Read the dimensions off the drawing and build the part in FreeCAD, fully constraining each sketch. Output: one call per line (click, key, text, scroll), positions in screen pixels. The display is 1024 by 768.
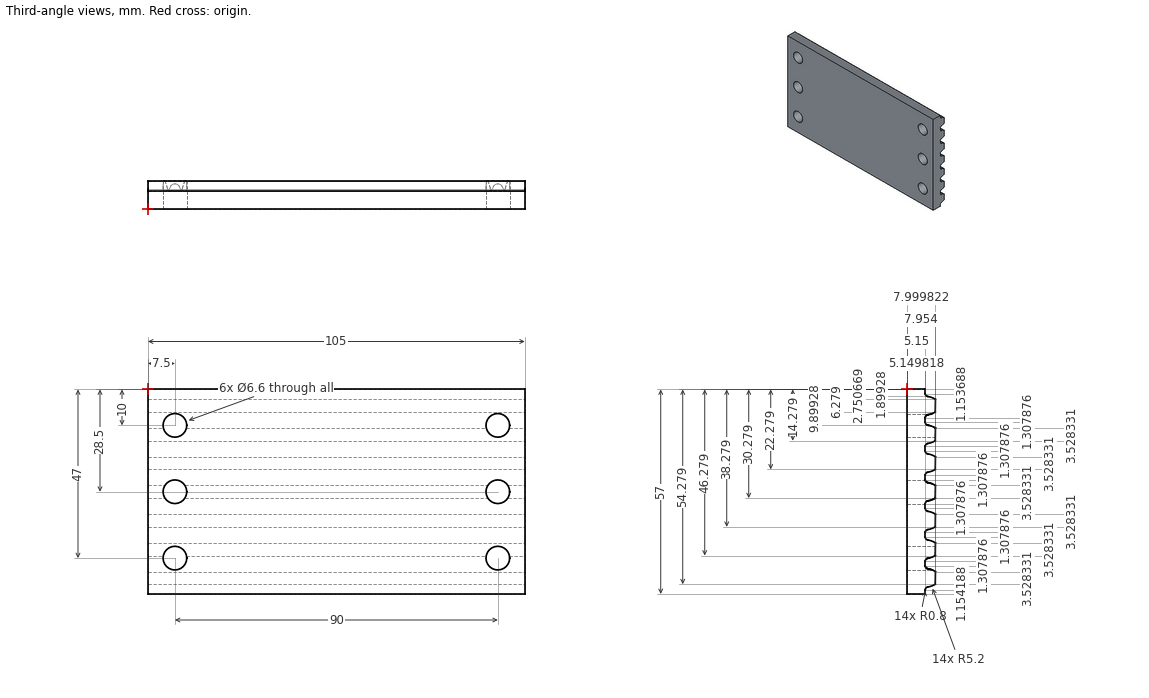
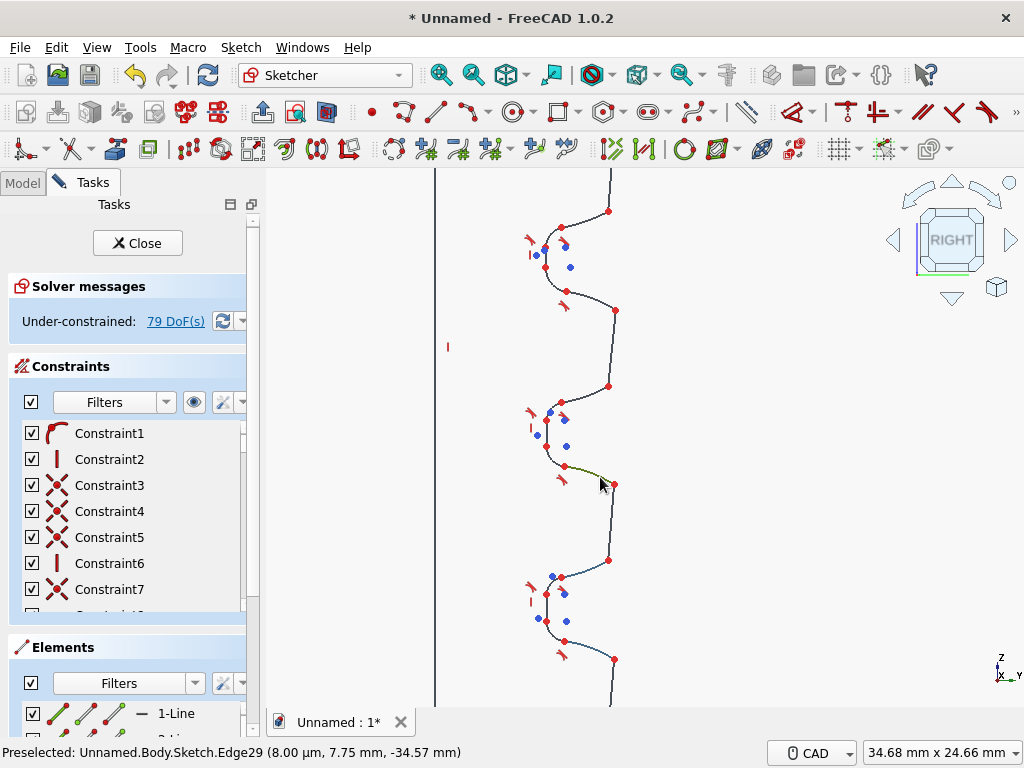
click(576, 400)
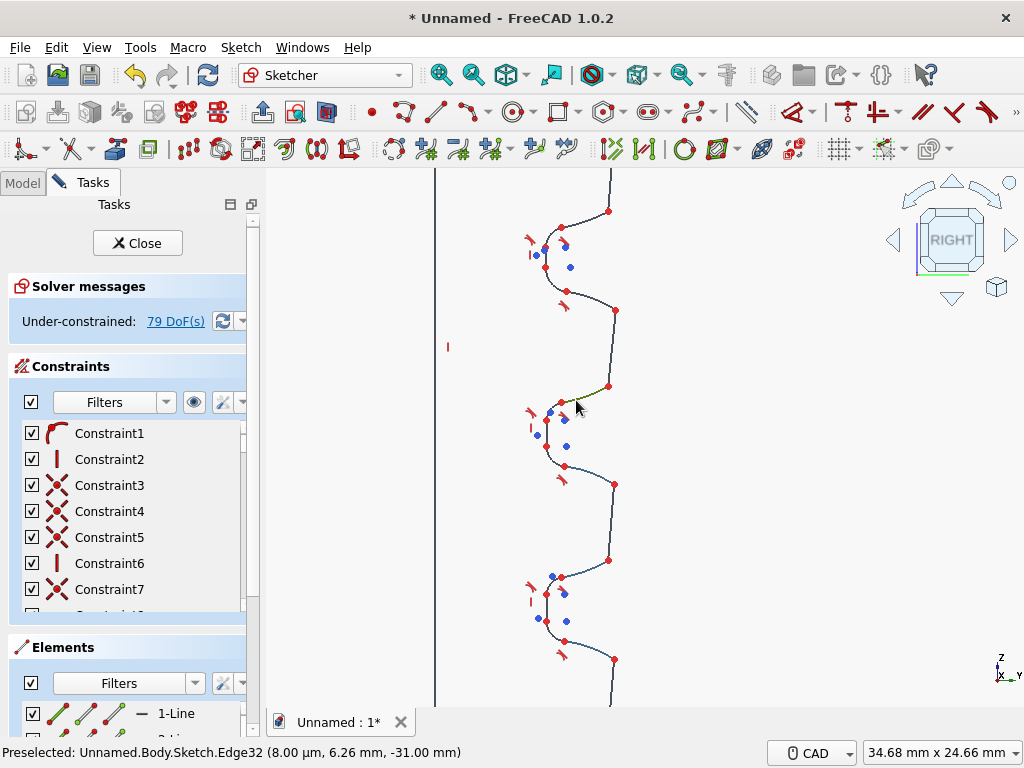
click(602, 302)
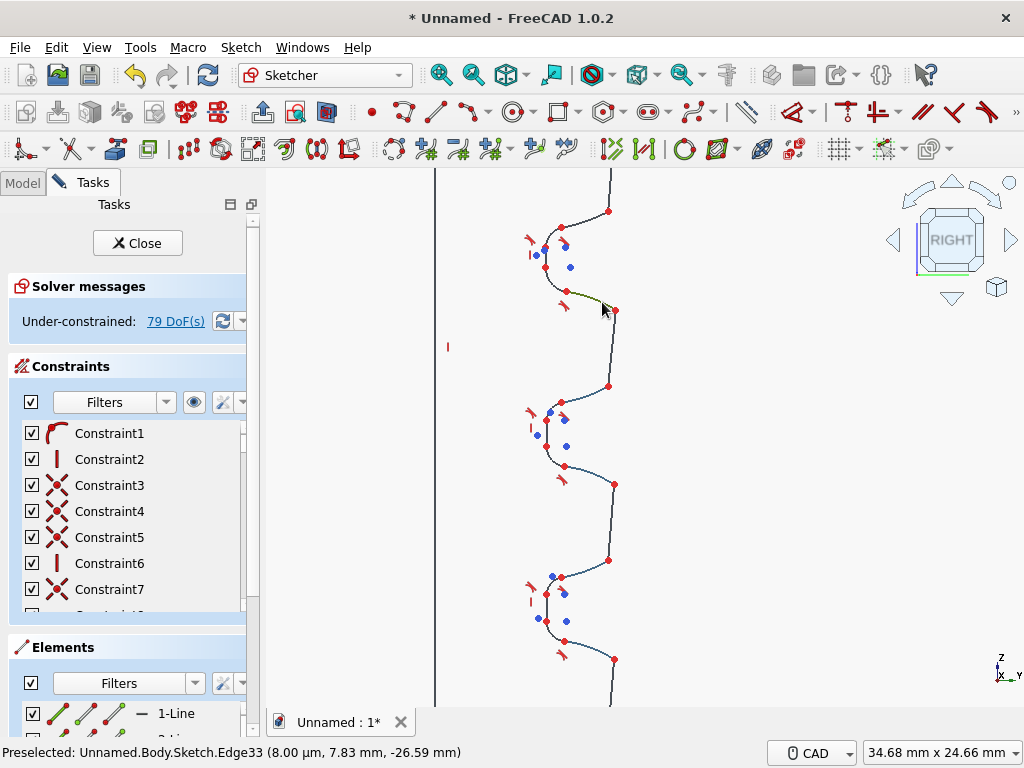
click(576, 224)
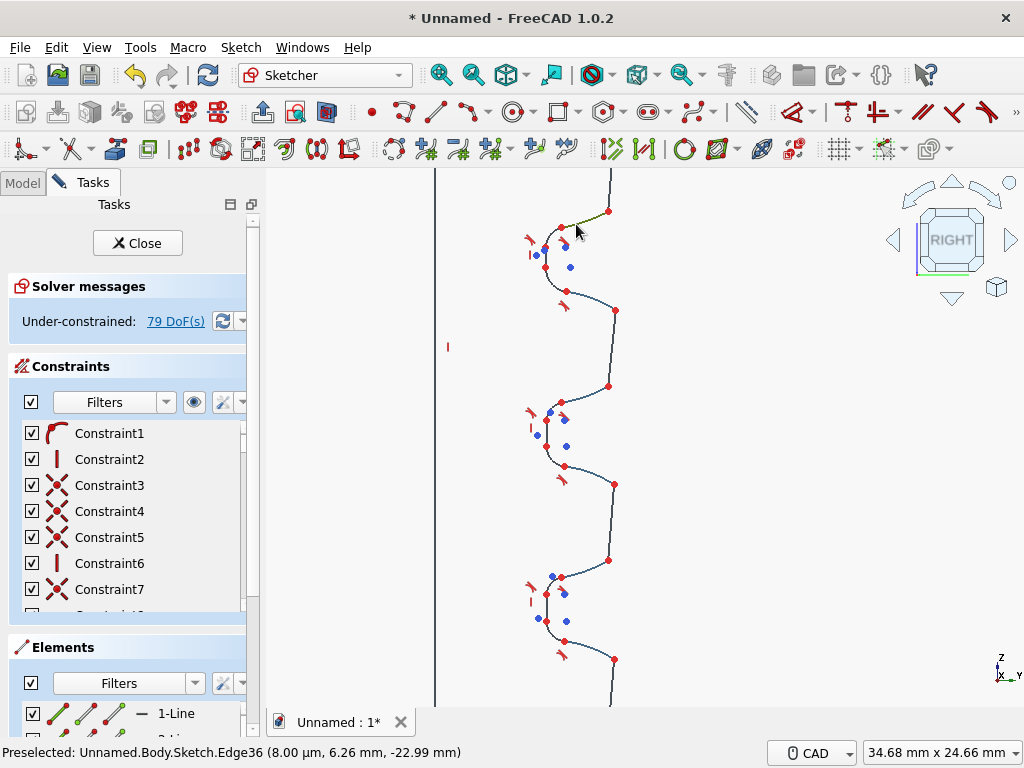
scroll(600, 477, down, 6)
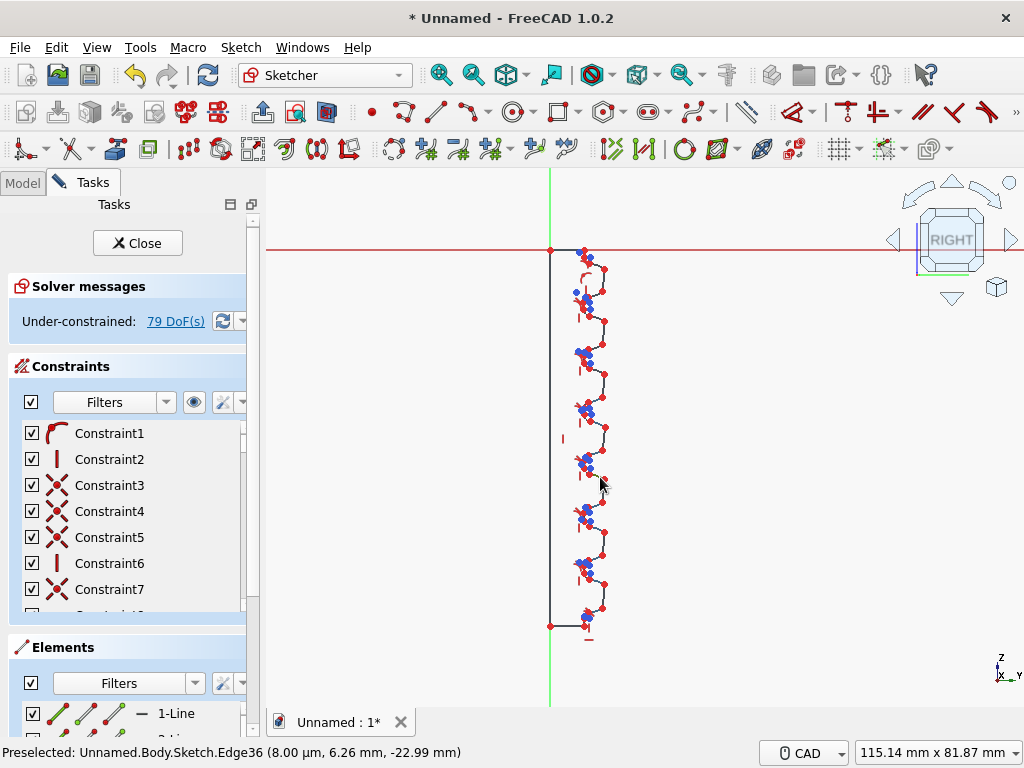
scroll(600, 372, up, 6)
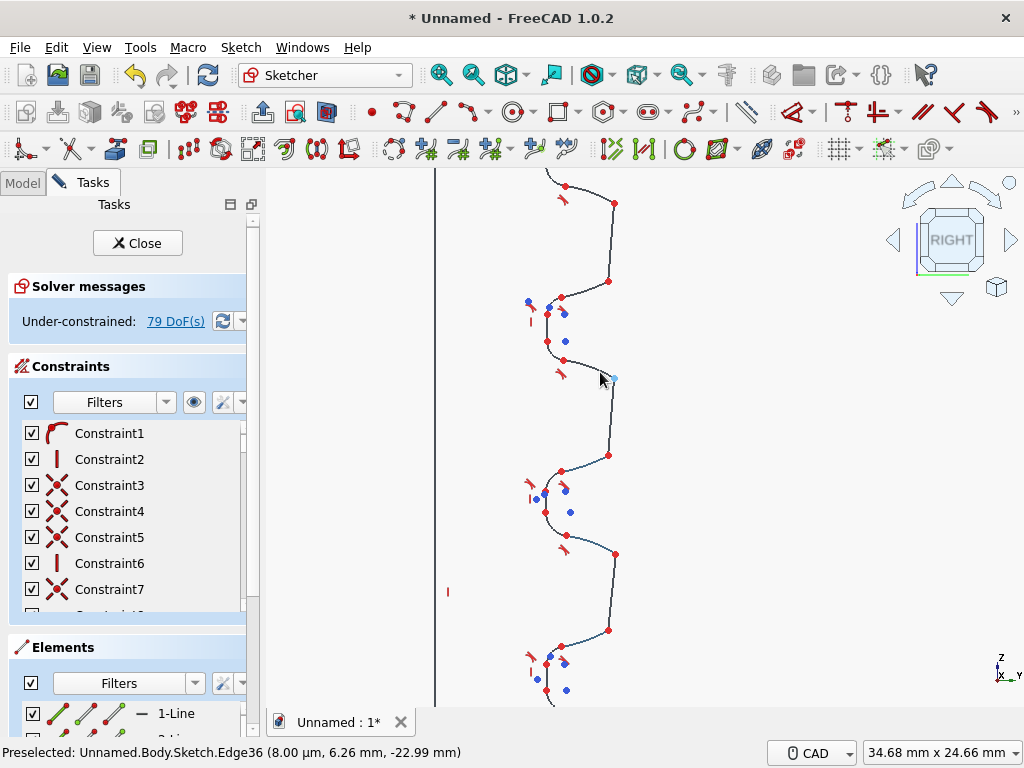
click(600, 371)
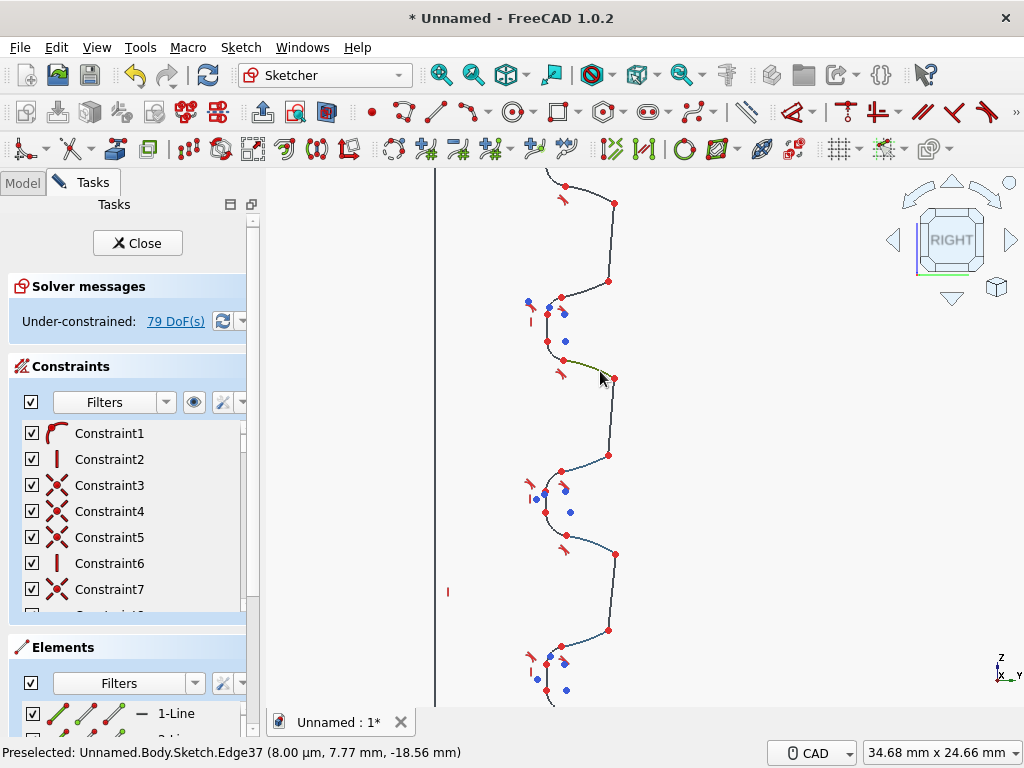
click(576, 294)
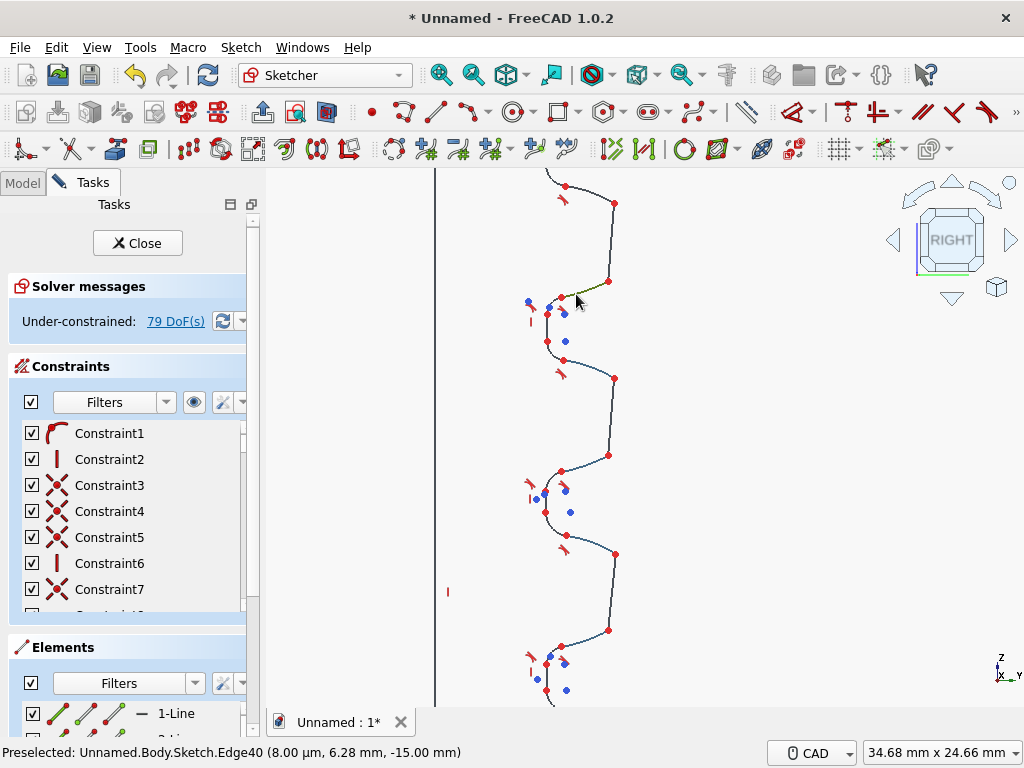
click(600, 196)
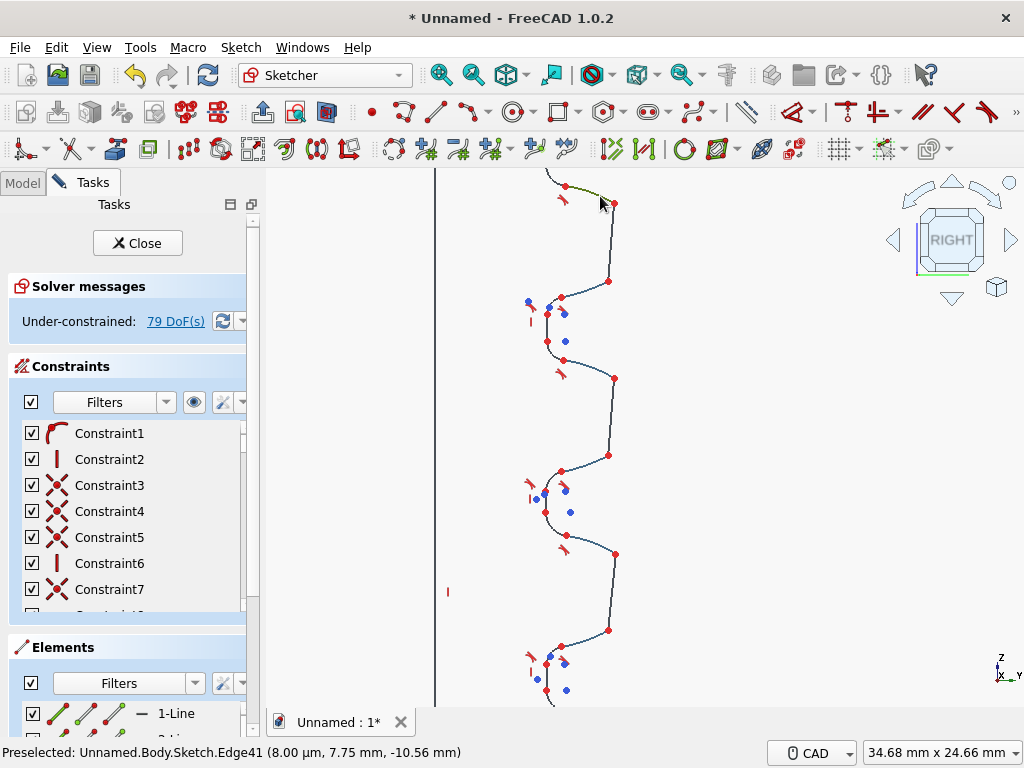
scroll(600, 372, down, 6)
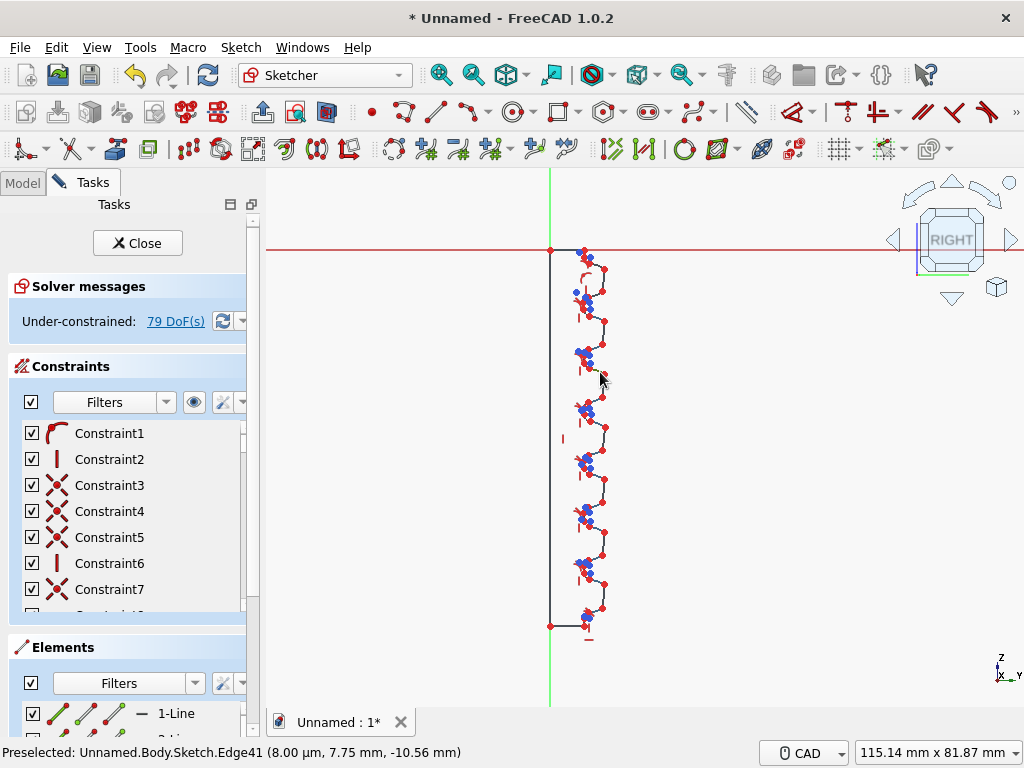
scroll(593, 296, up, 6)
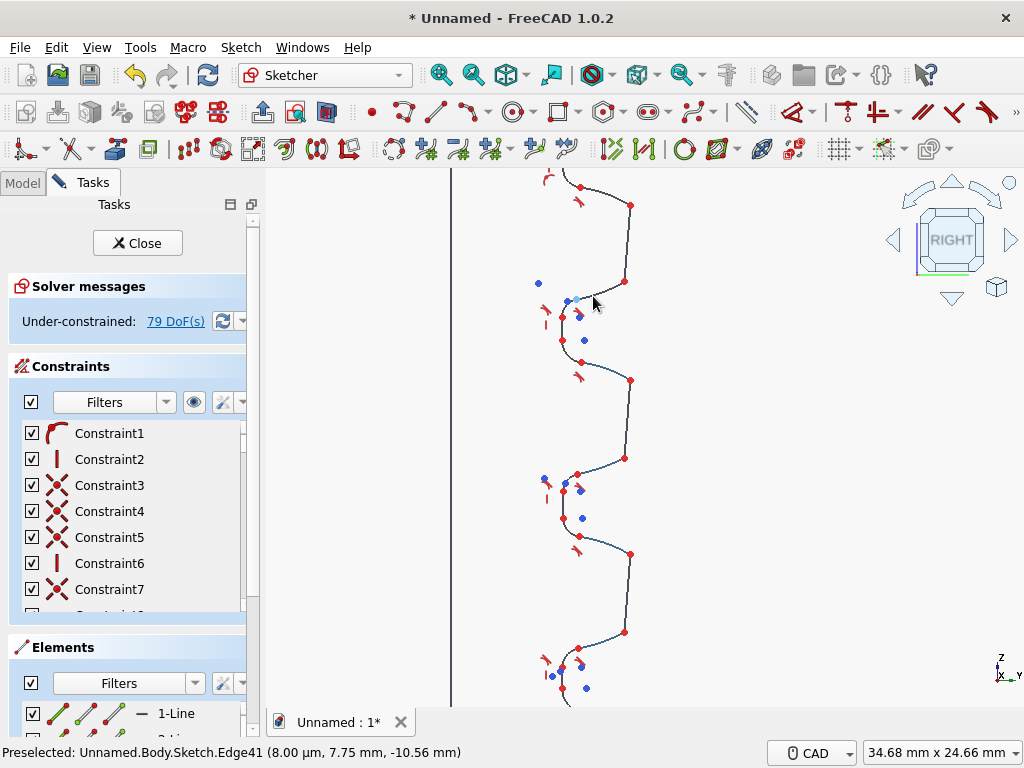
click(592, 296)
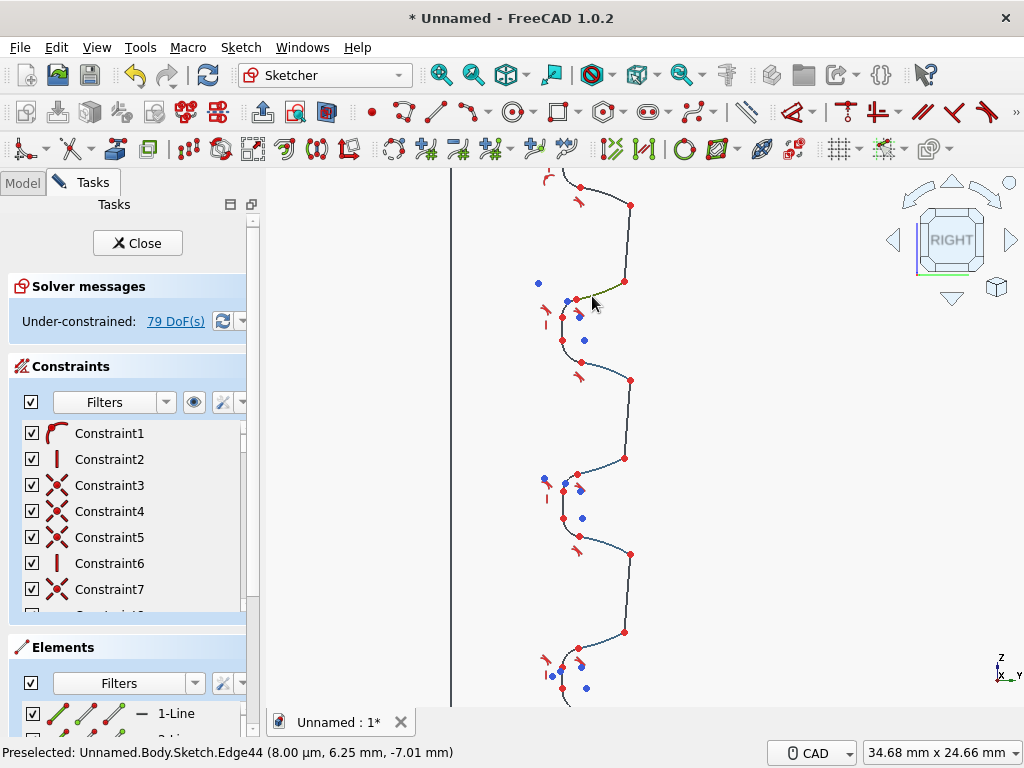
click(616, 198)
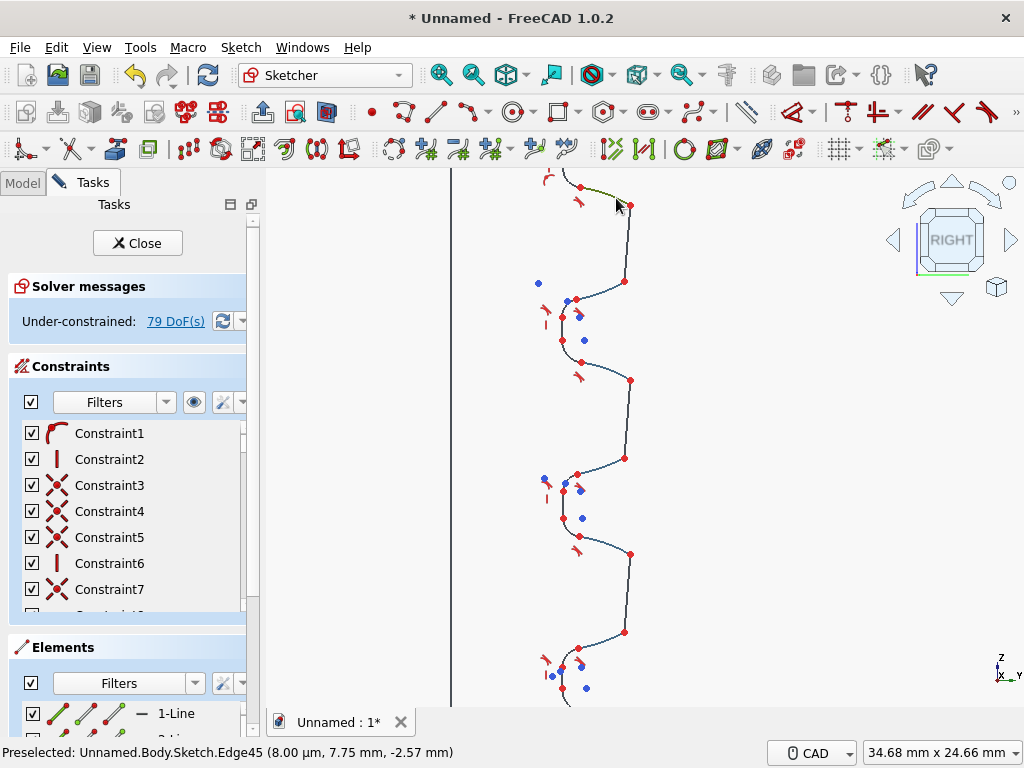
key(e)